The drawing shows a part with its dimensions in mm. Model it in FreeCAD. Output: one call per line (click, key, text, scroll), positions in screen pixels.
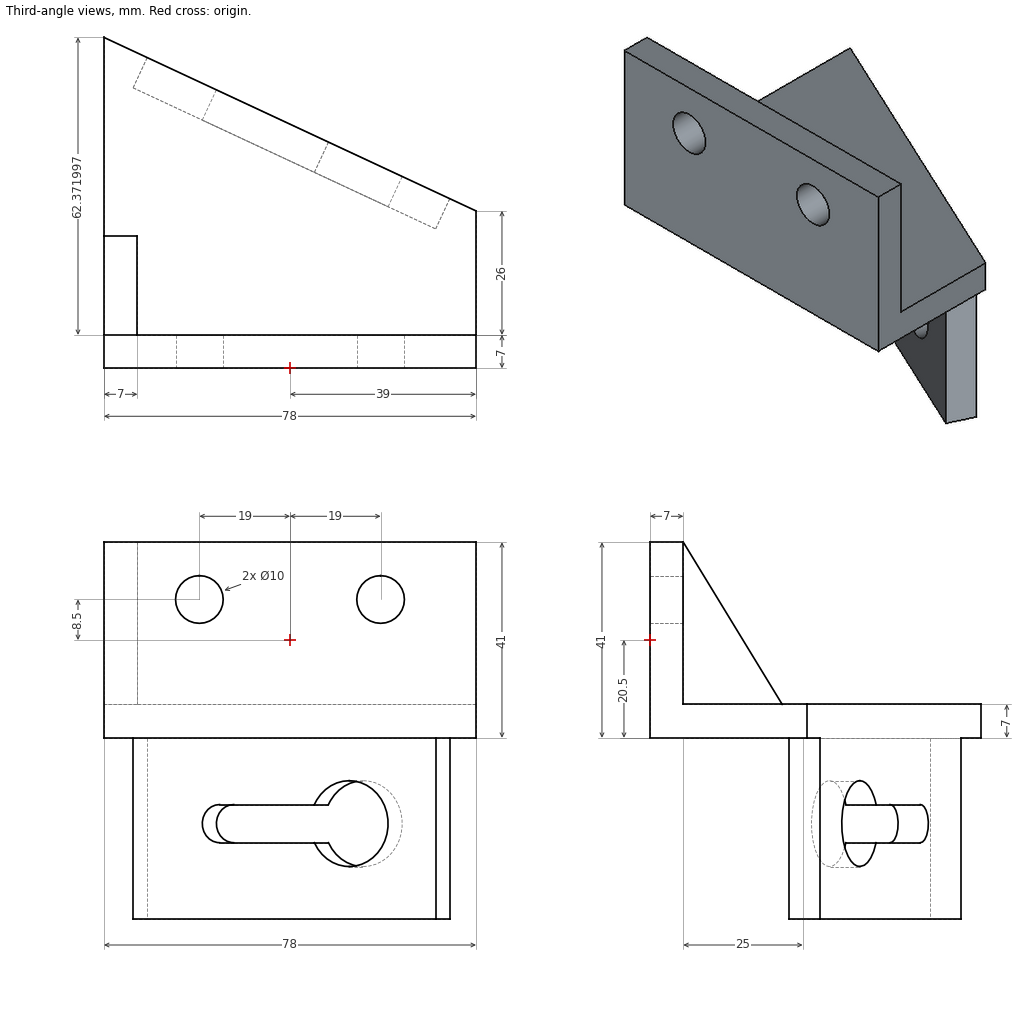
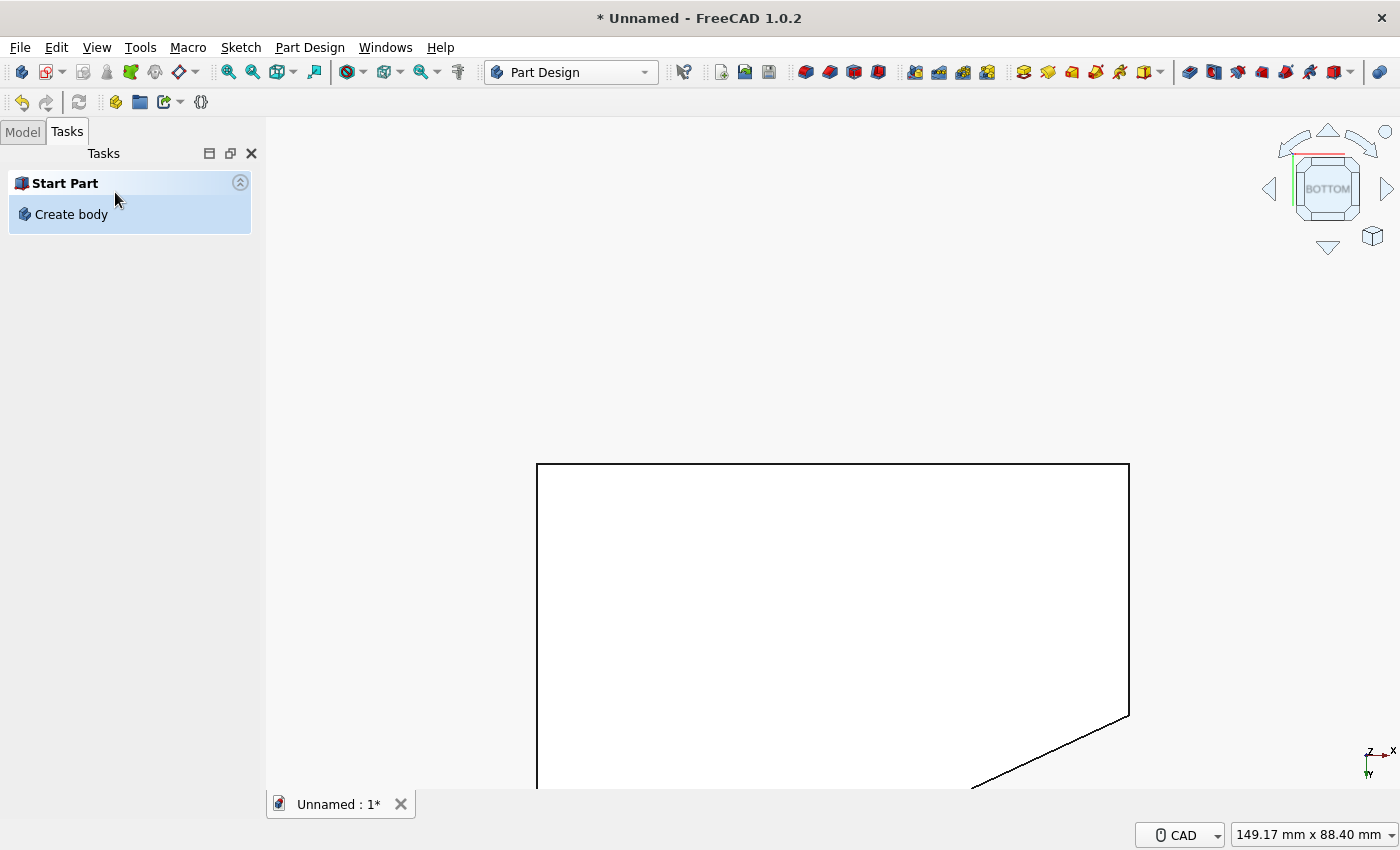
click(230, 72)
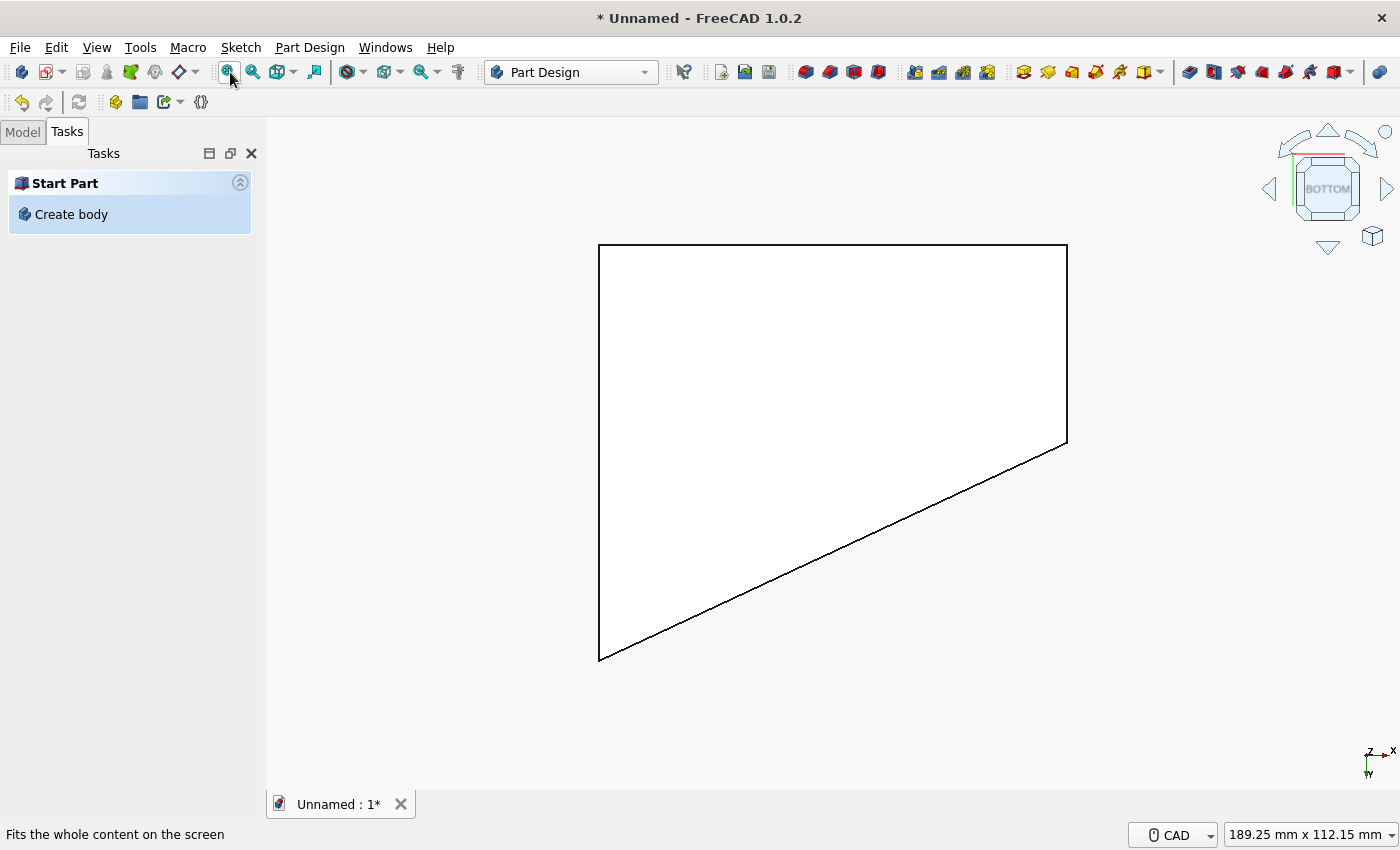
key(4)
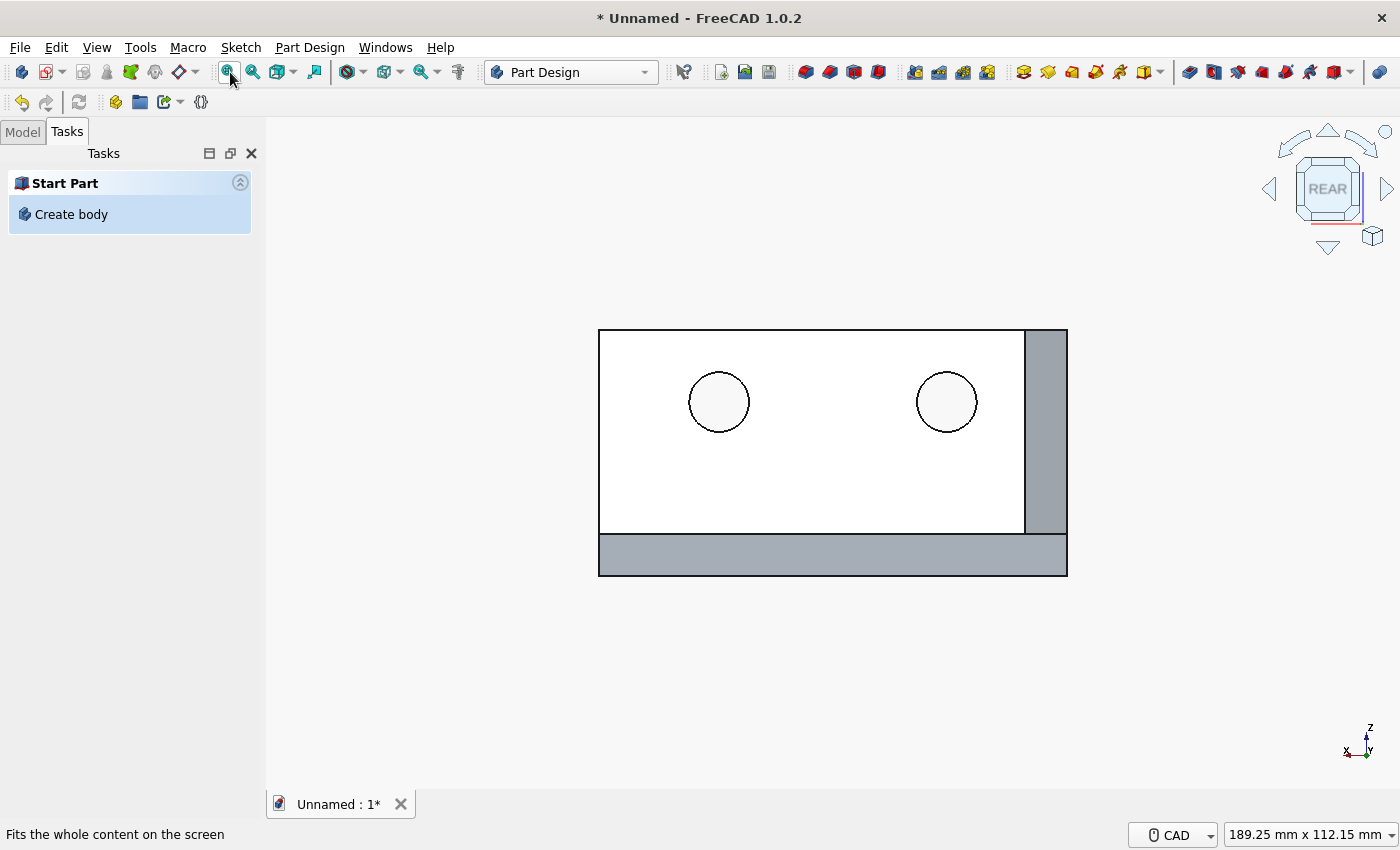
click(230, 72)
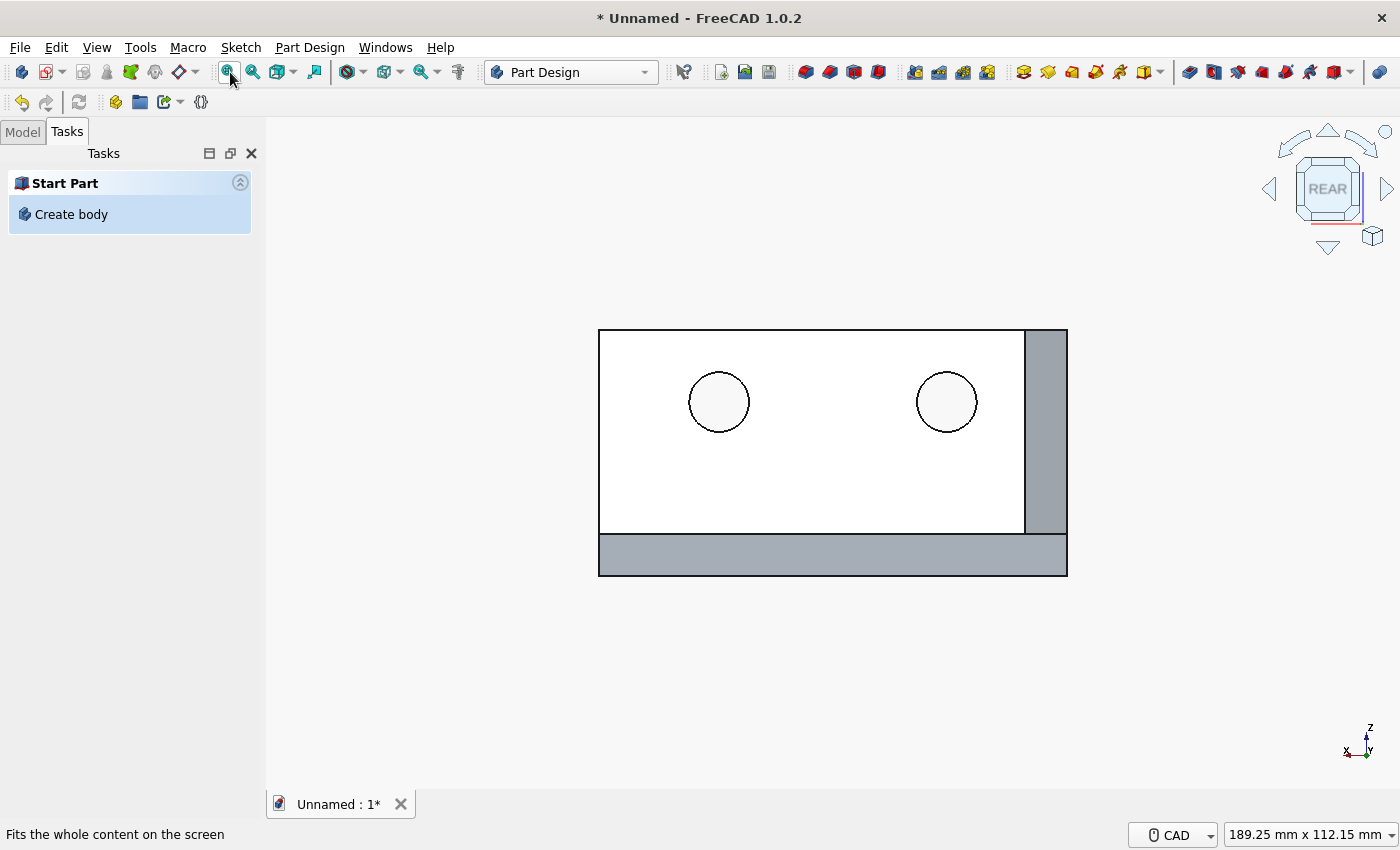
click(633, 554)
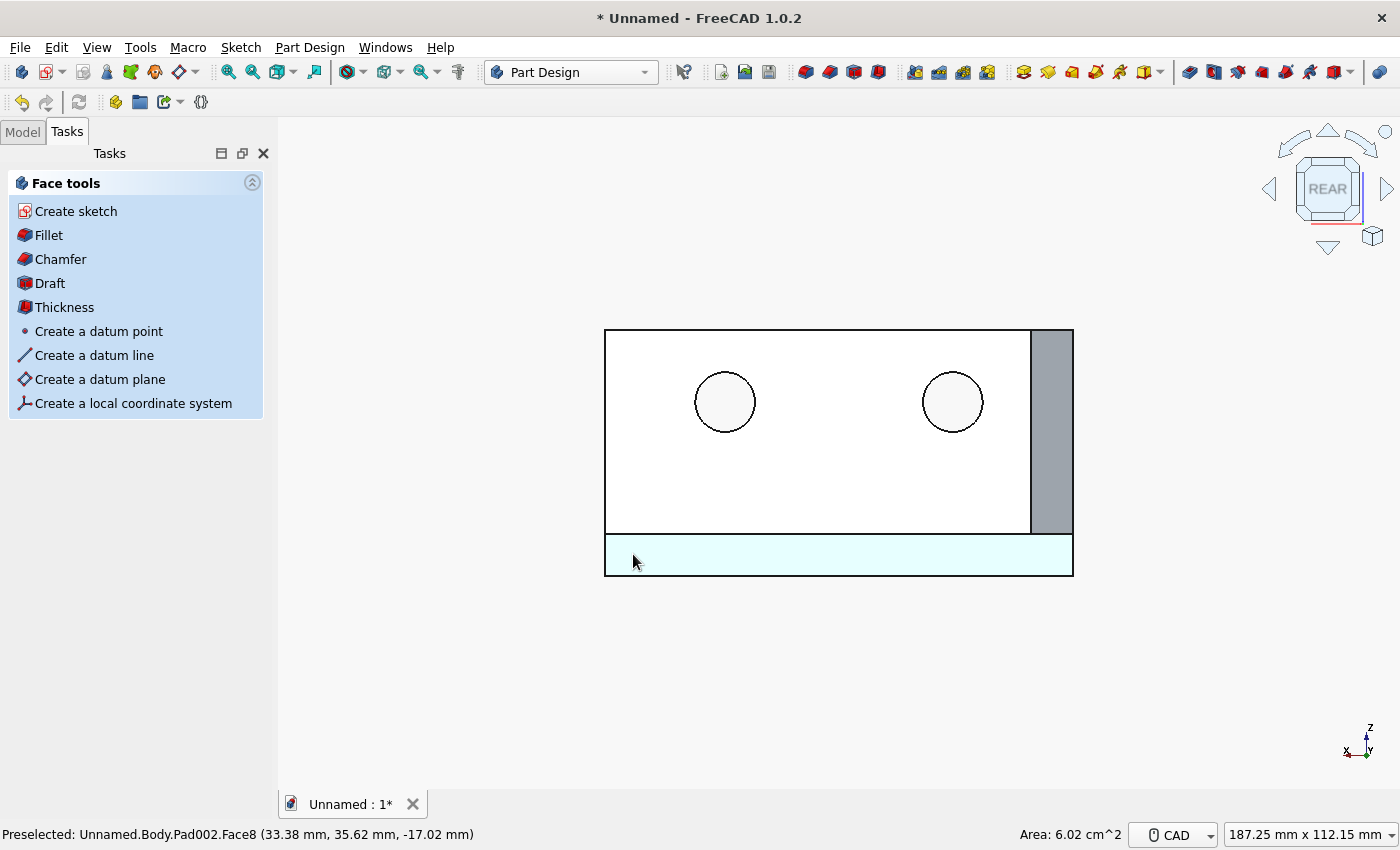
click(46, 72)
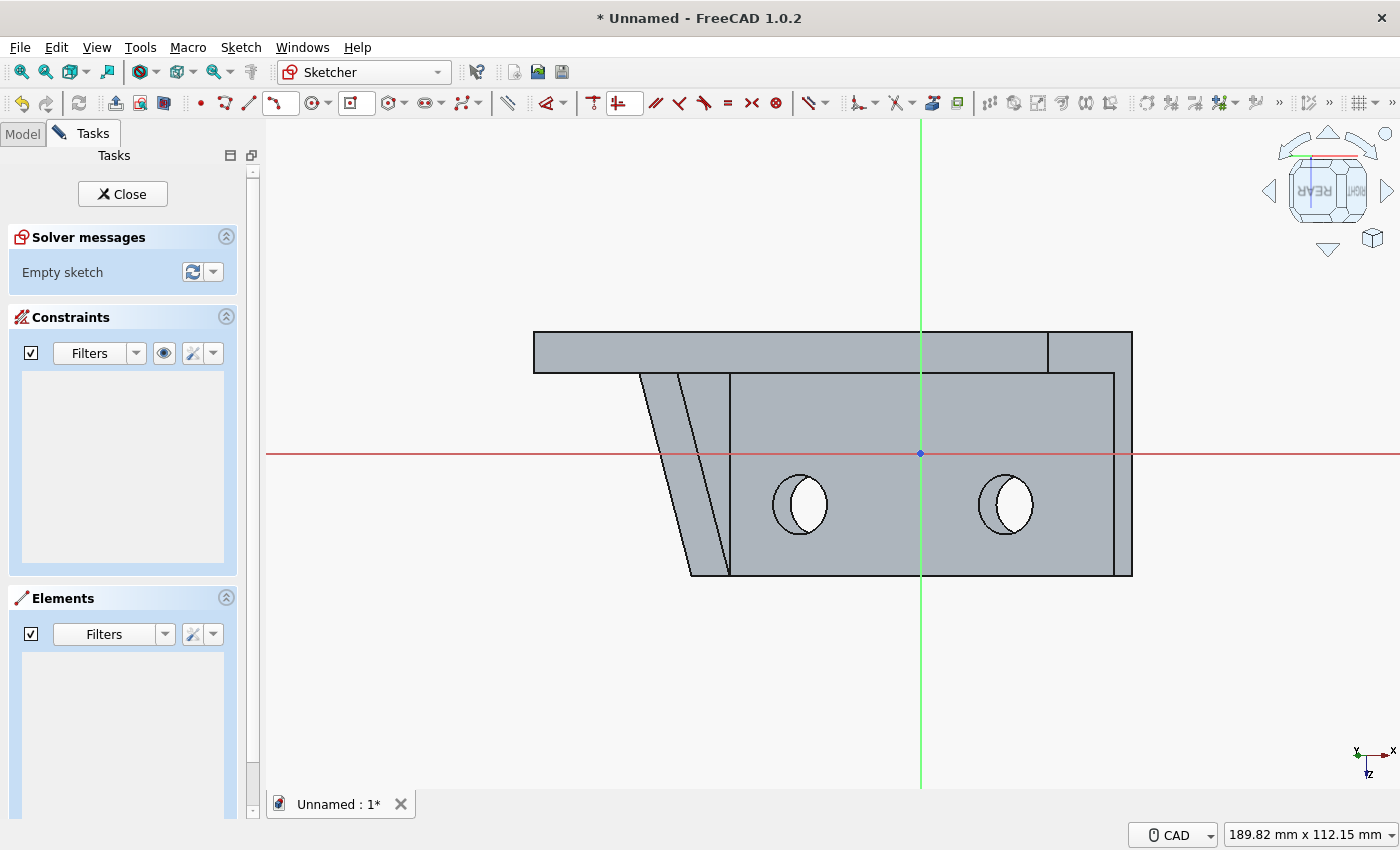
scroll(590, 761, down, 1)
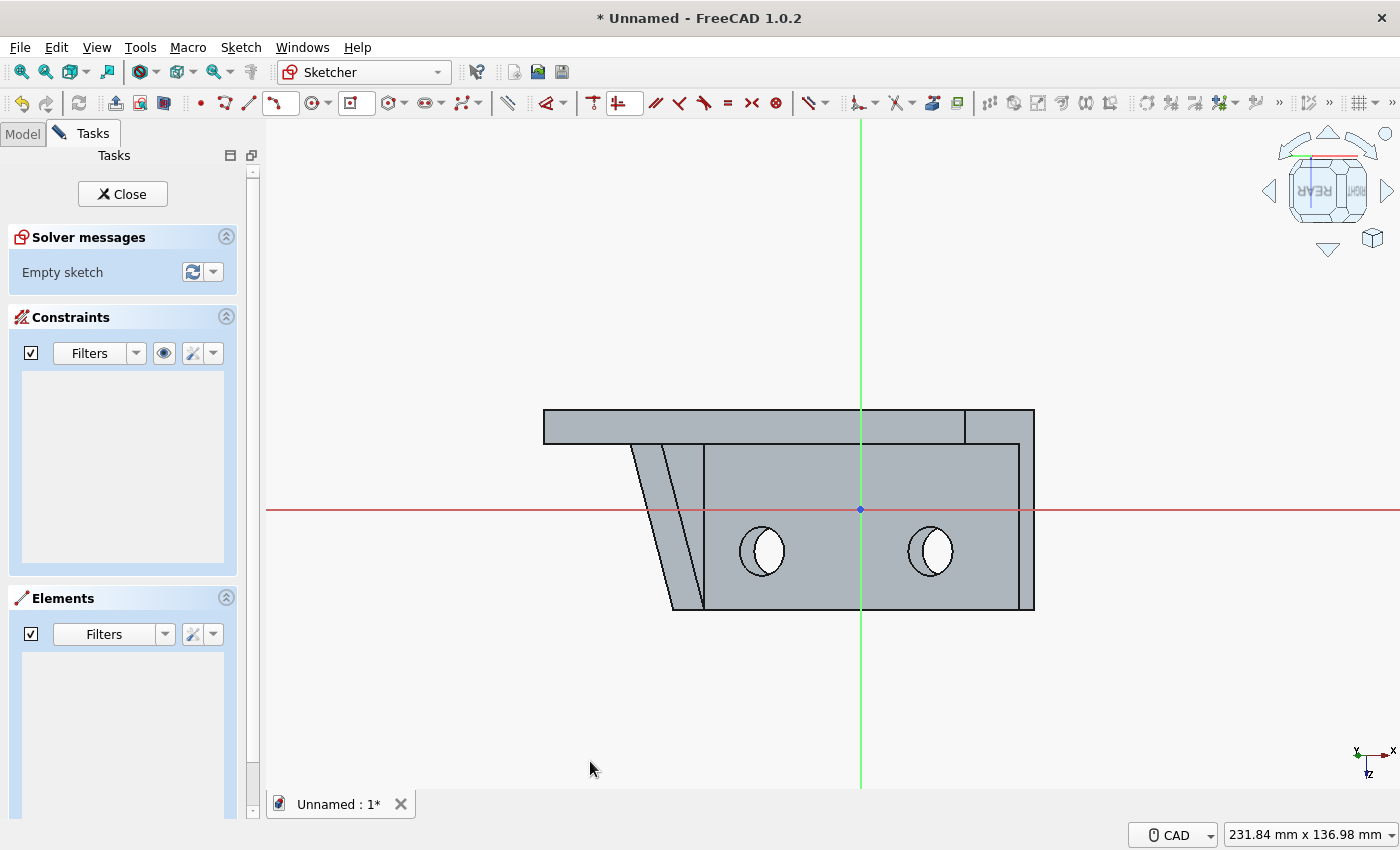
scroll(765, 189, up, 2)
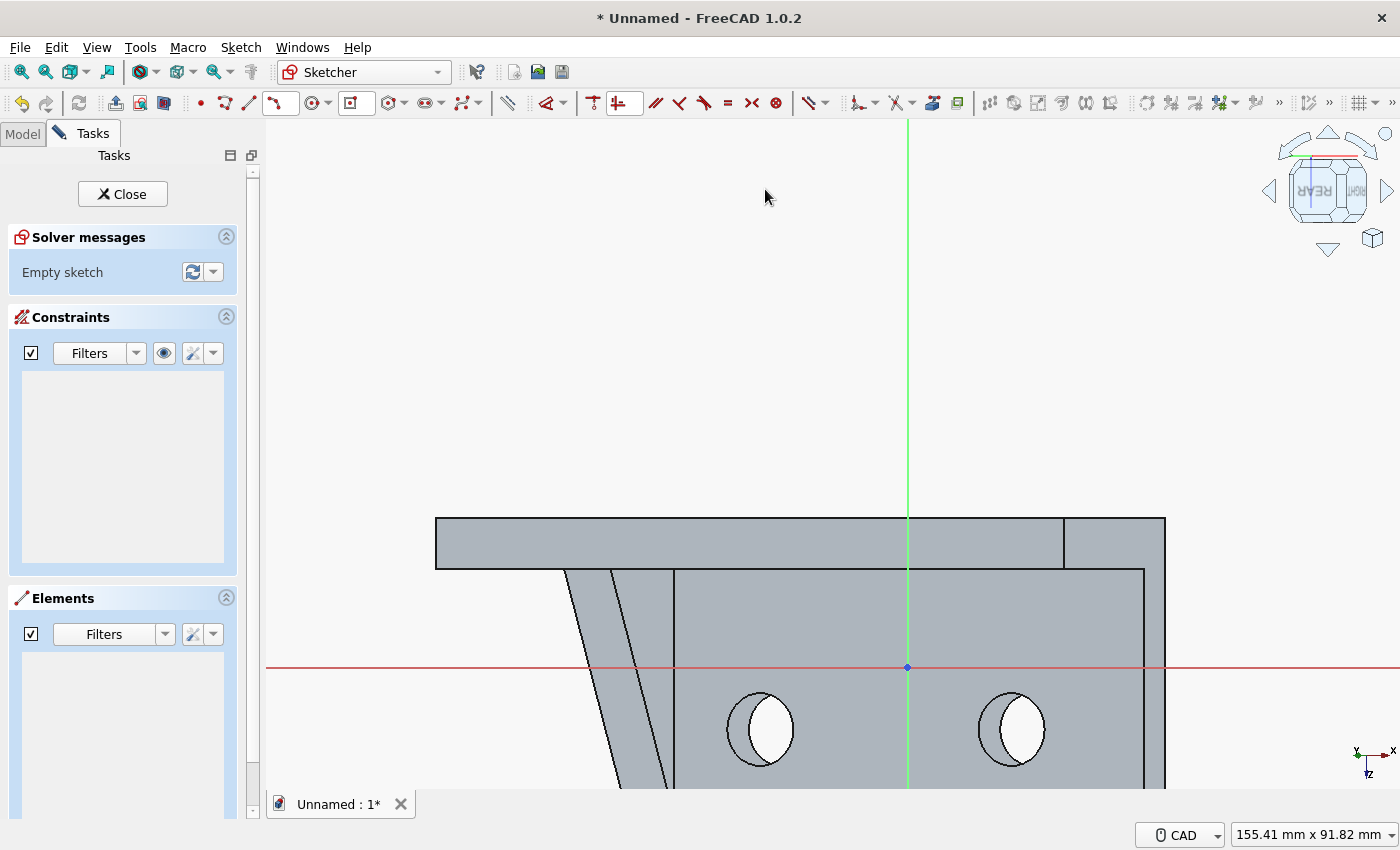
key(g)
key(r)